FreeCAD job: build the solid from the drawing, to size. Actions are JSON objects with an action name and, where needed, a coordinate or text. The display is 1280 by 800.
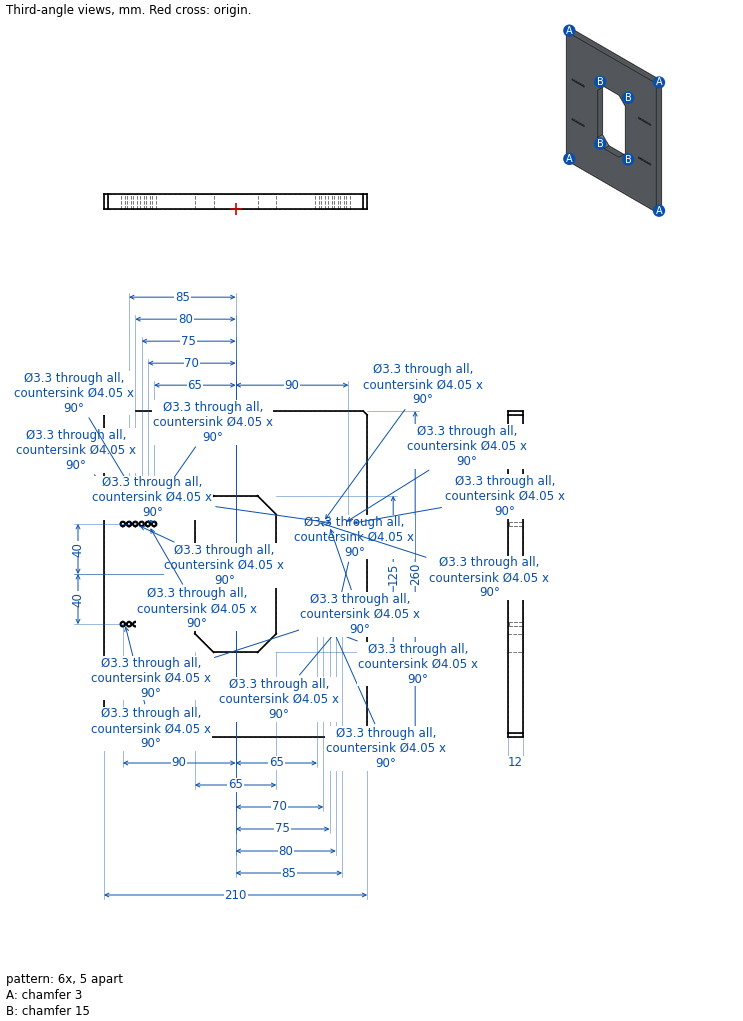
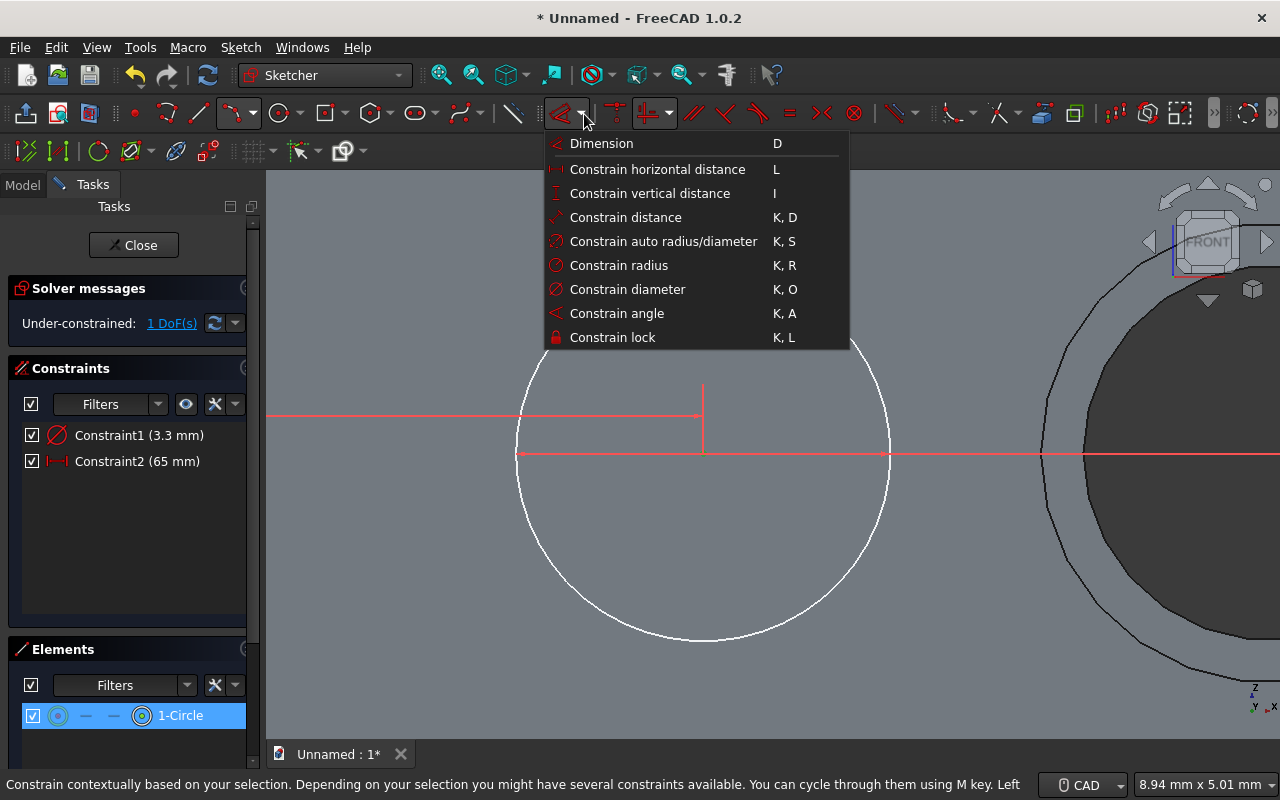
{"action": "left_click", "coordinate": [697, 193]}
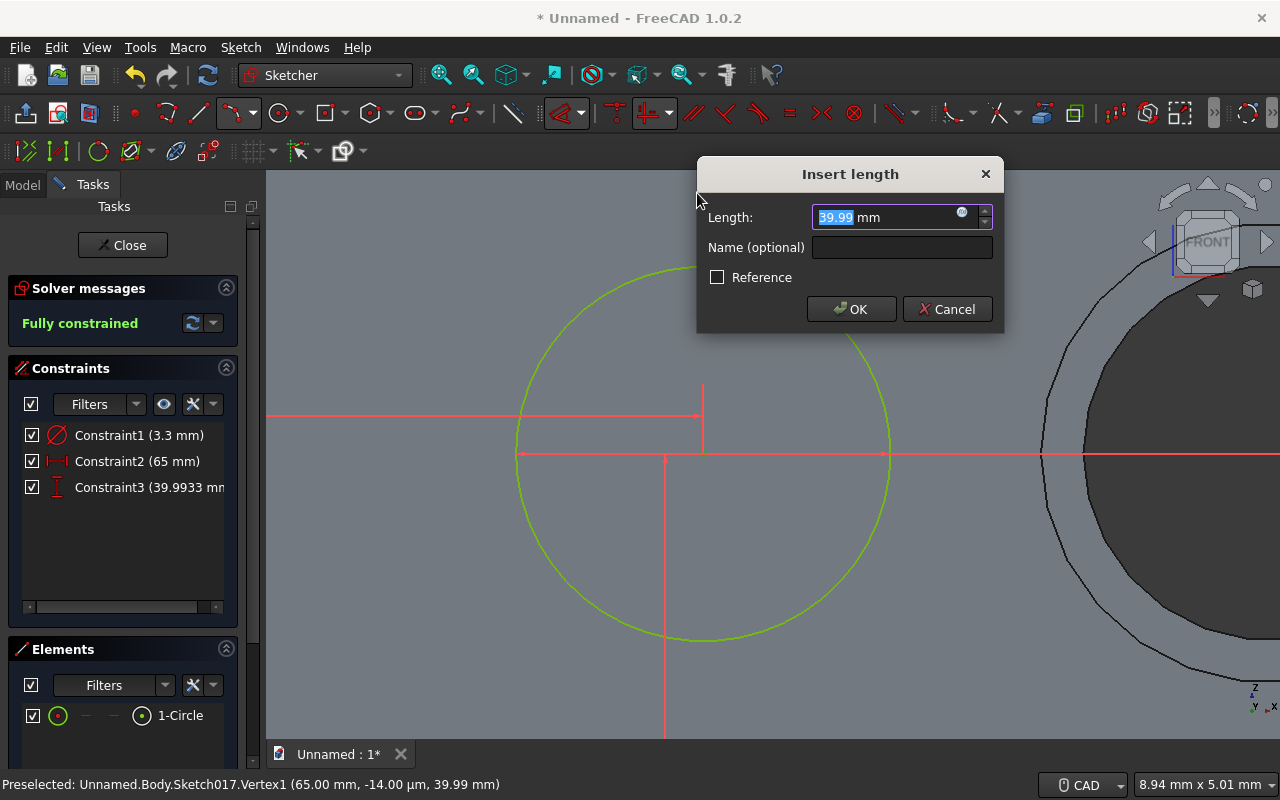
{"action": "type", "text": "40"}
{"action": "key", "text": "Return"}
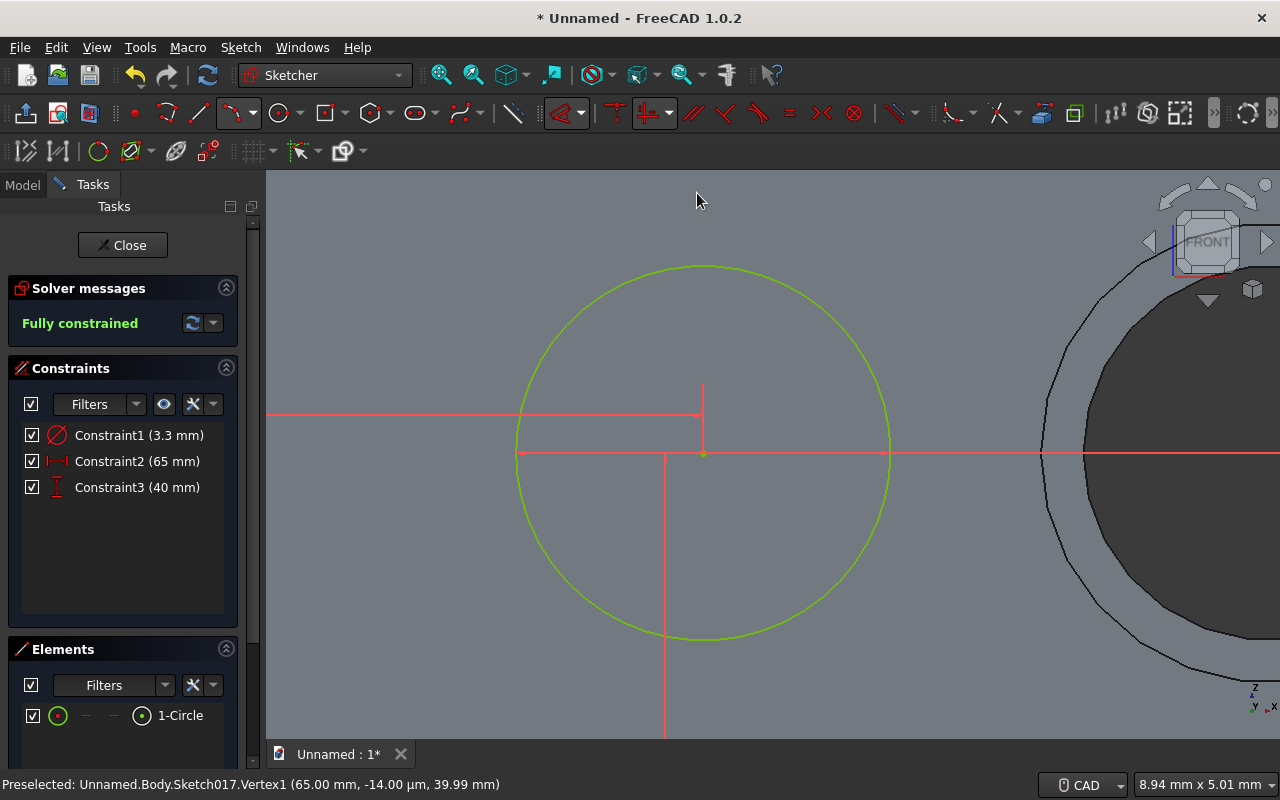
{"action": "left_click", "coordinate": [123, 245]}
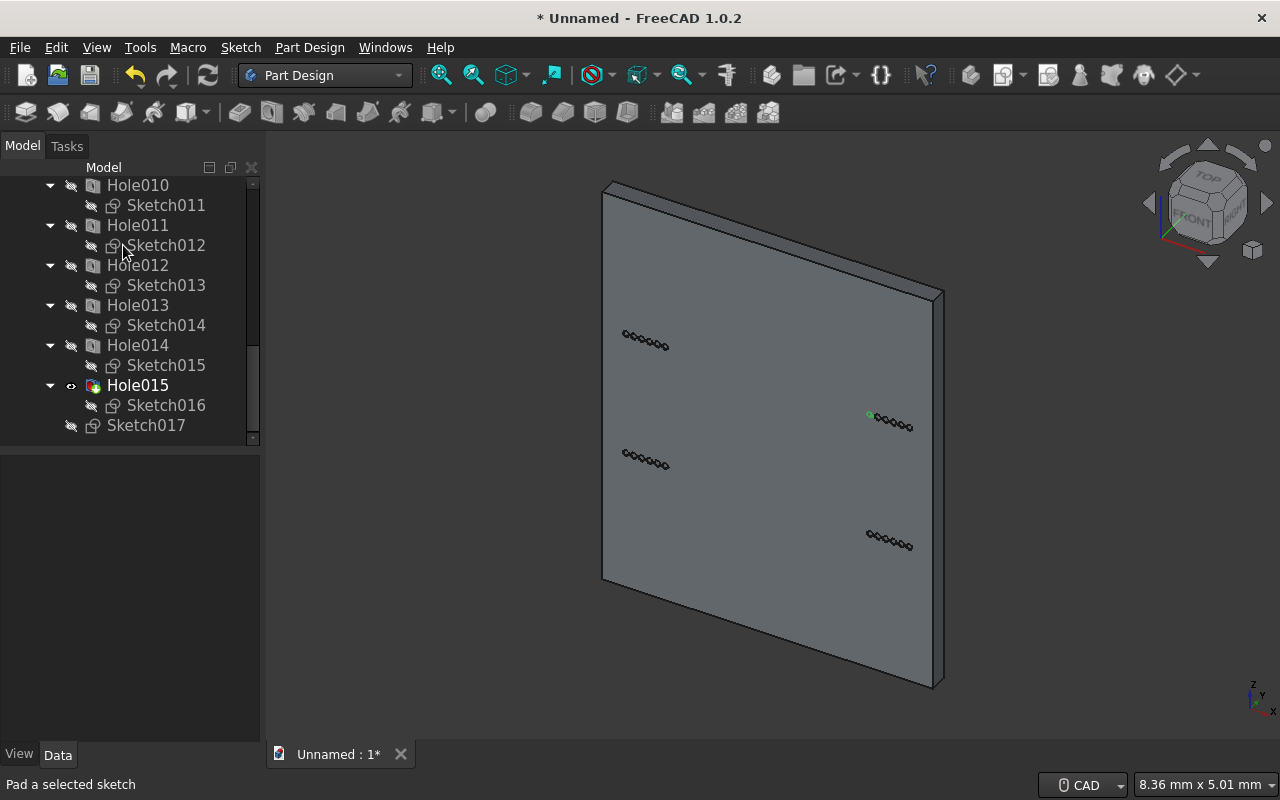
{"action": "left_click", "coordinate": [272, 112]}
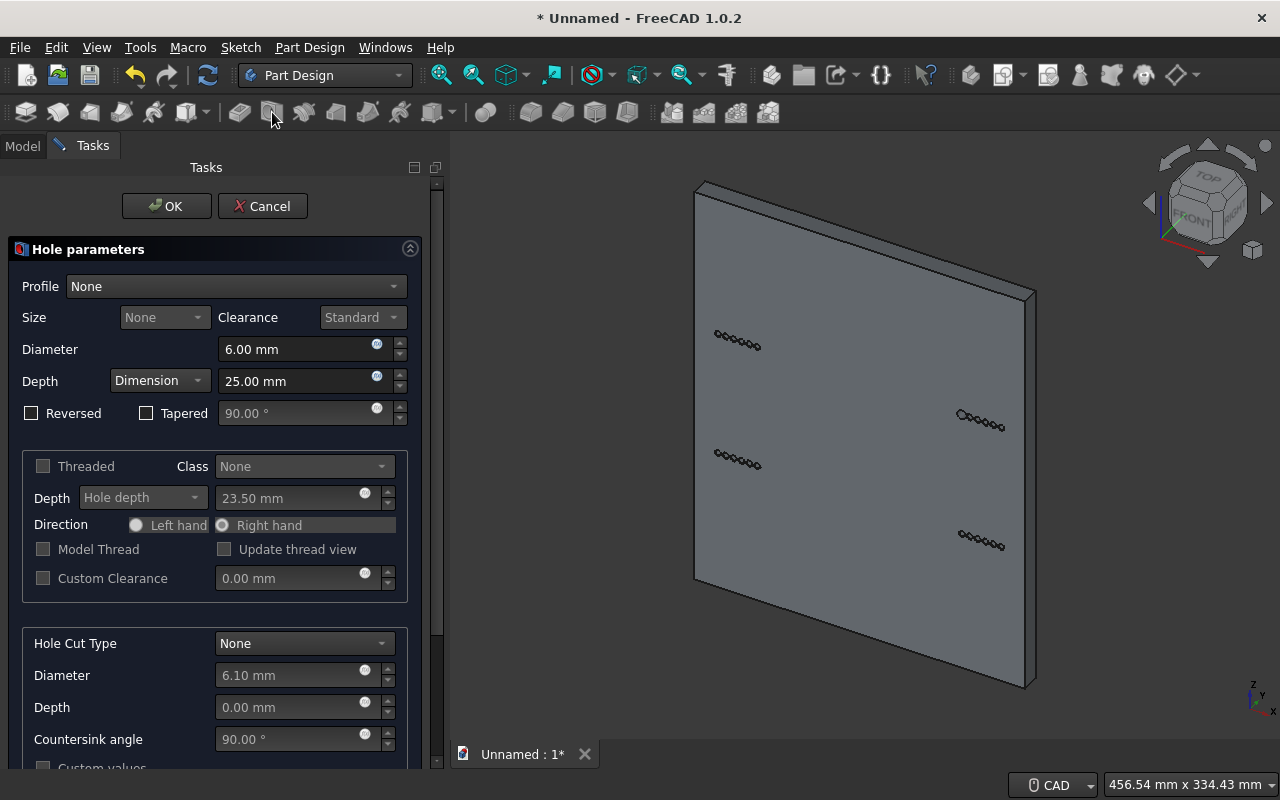
{"action": "triple_click", "coordinate": [305, 349]}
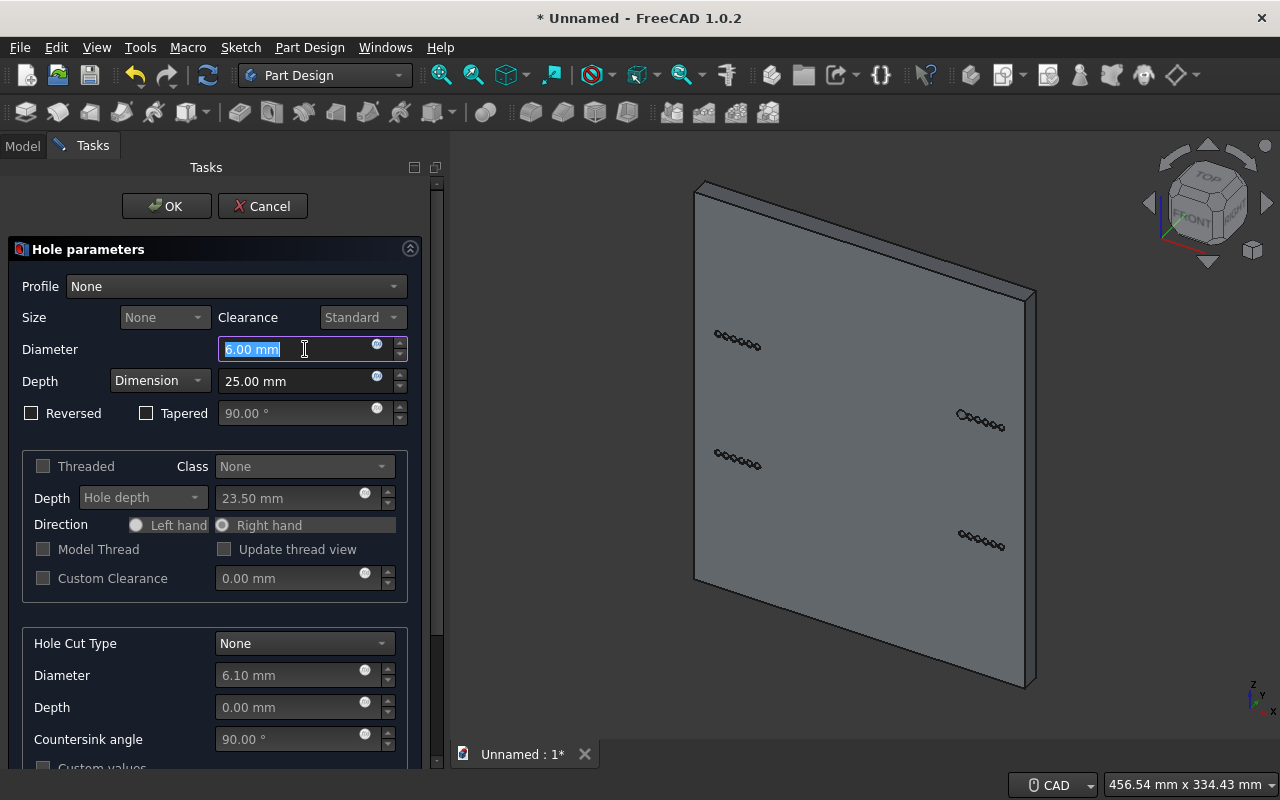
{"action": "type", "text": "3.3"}
{"action": "key", "text": "Tab"}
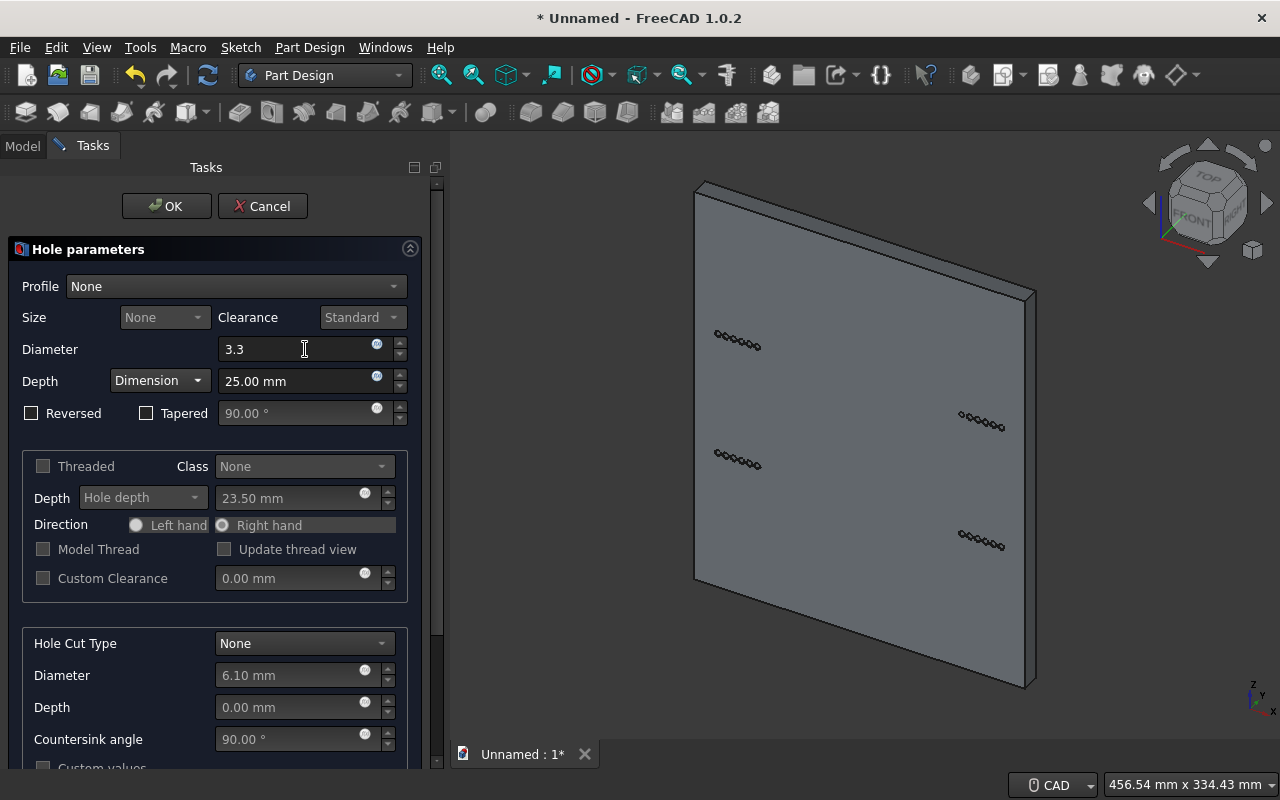
{"action": "left_click", "coordinate": [161, 380]}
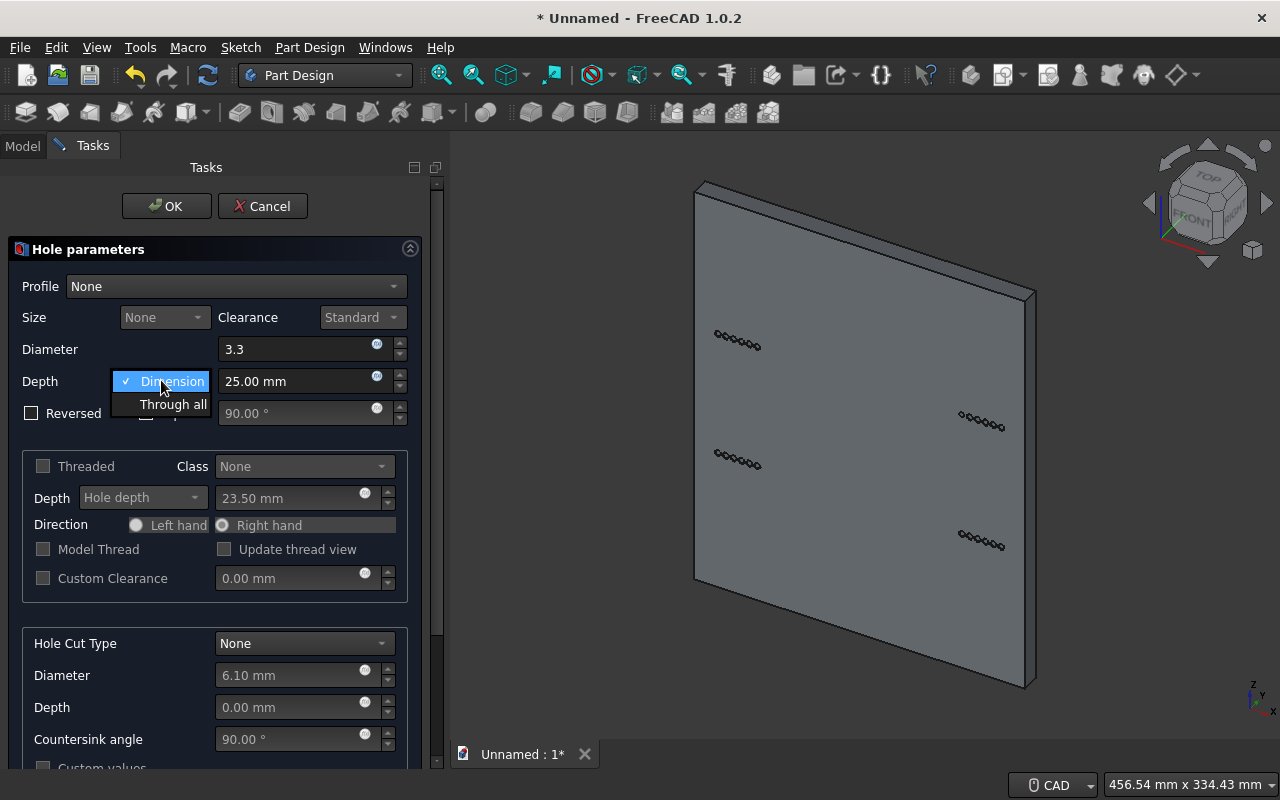
{"action": "left_click", "coordinate": [160, 404]}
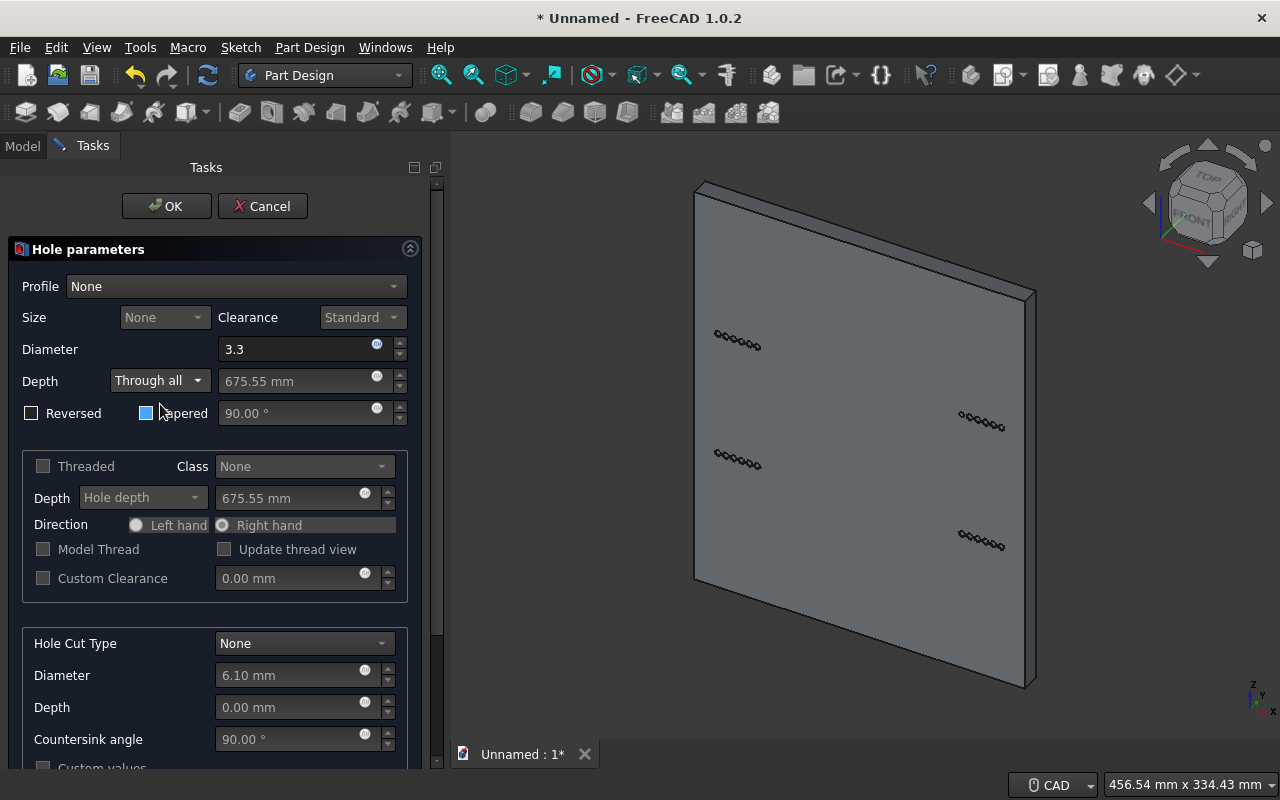
{"action": "left_click", "coordinate": [306, 644]}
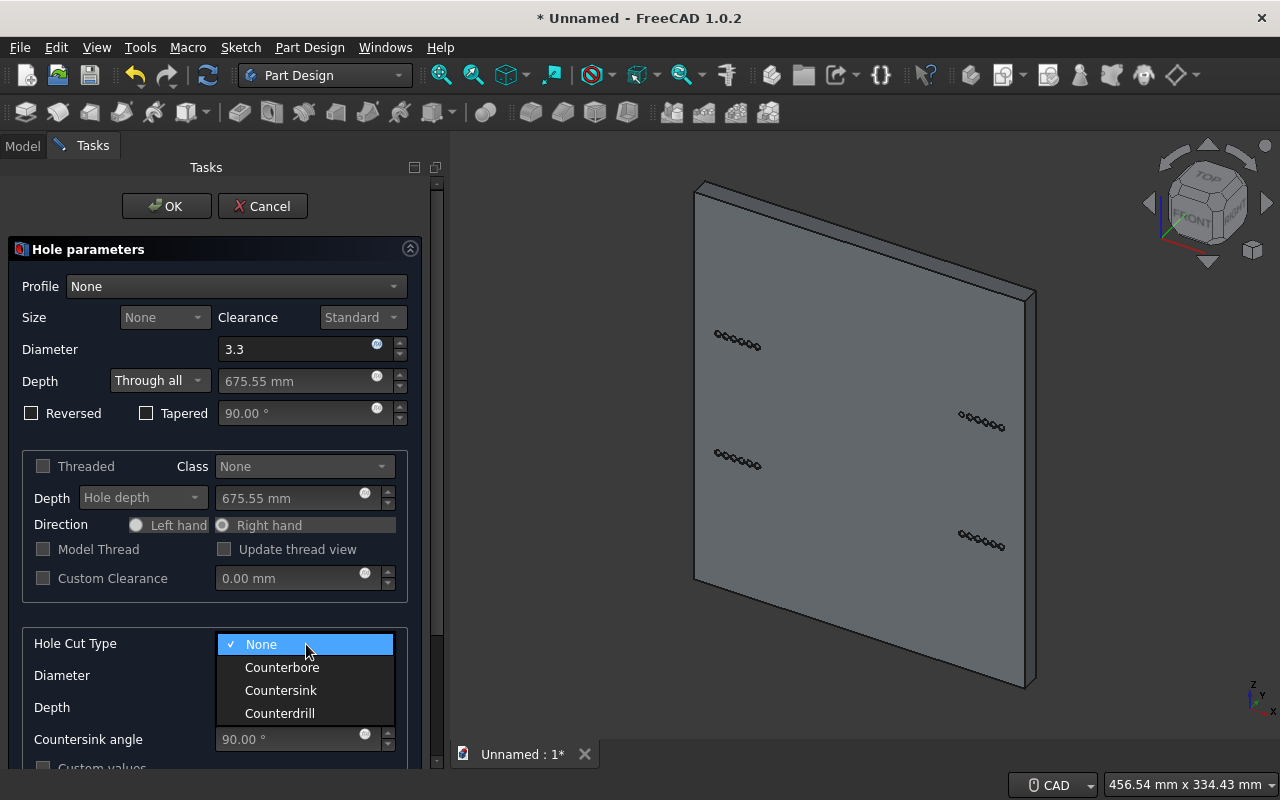
{"action": "left_click", "coordinate": [304, 690]}